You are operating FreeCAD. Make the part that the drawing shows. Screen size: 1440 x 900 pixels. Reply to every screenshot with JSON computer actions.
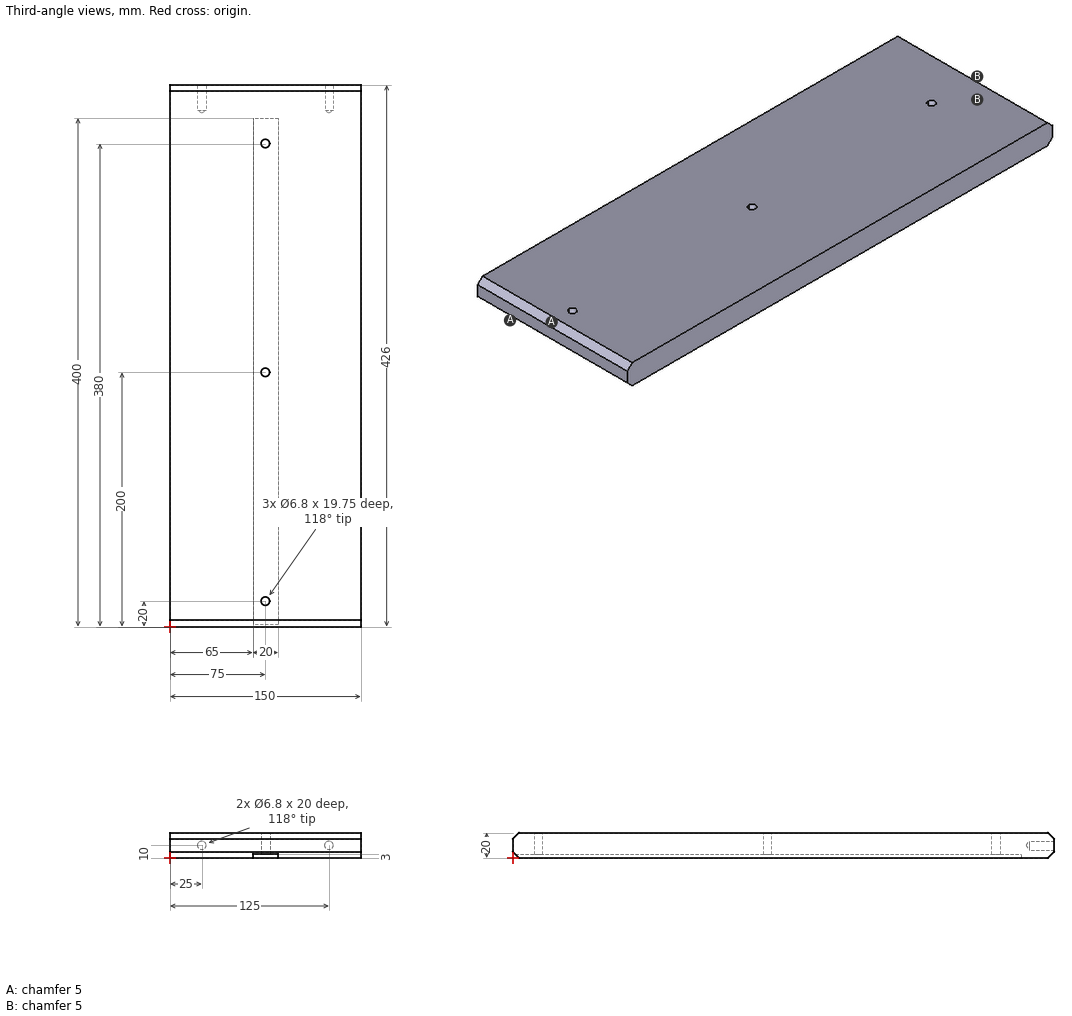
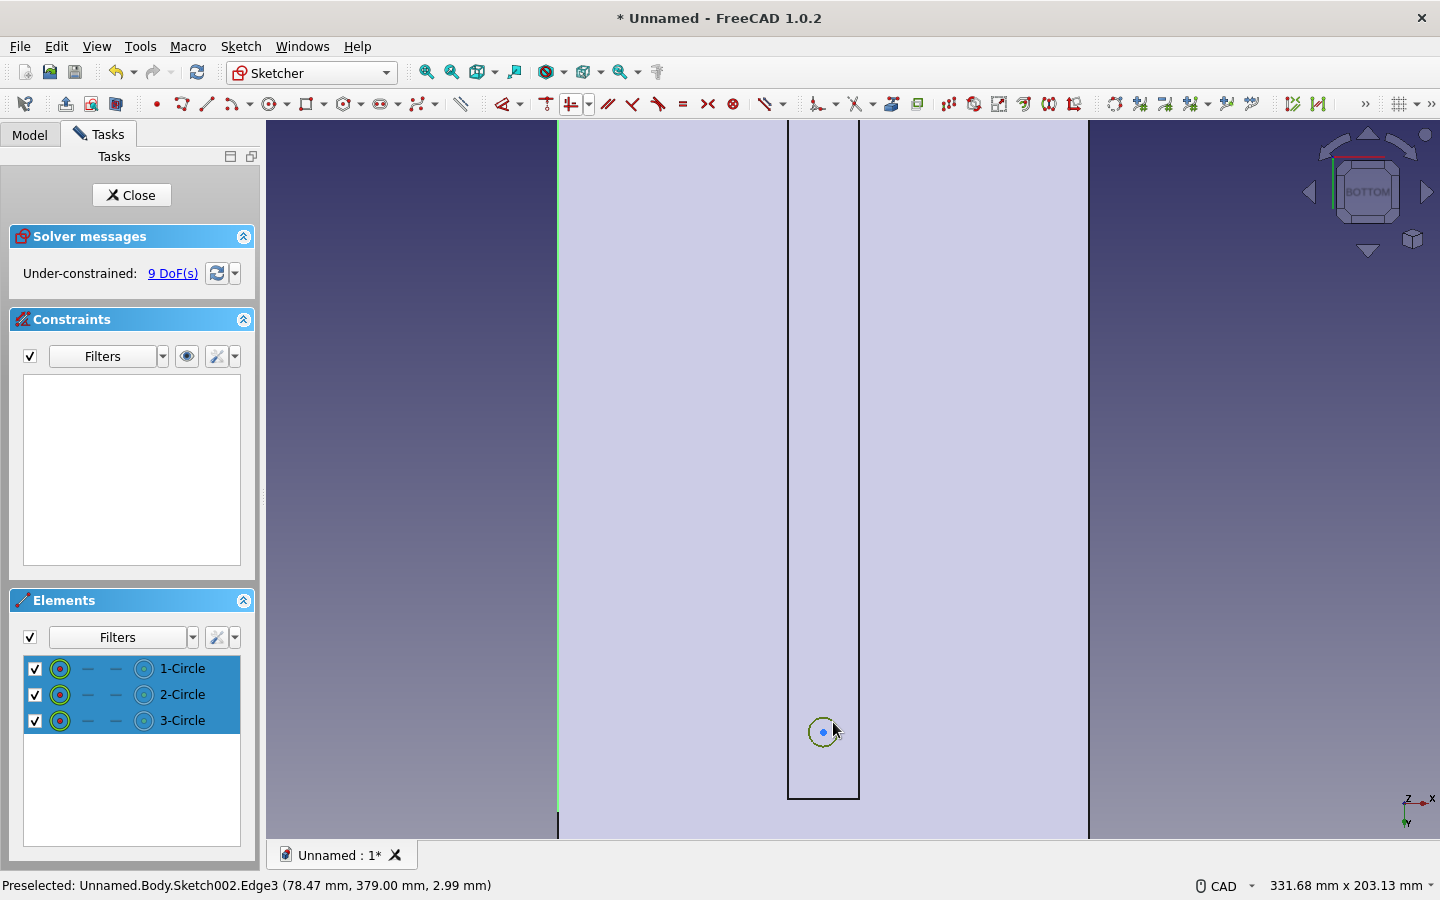
{"action": "left_click", "coordinate": [683, 104]}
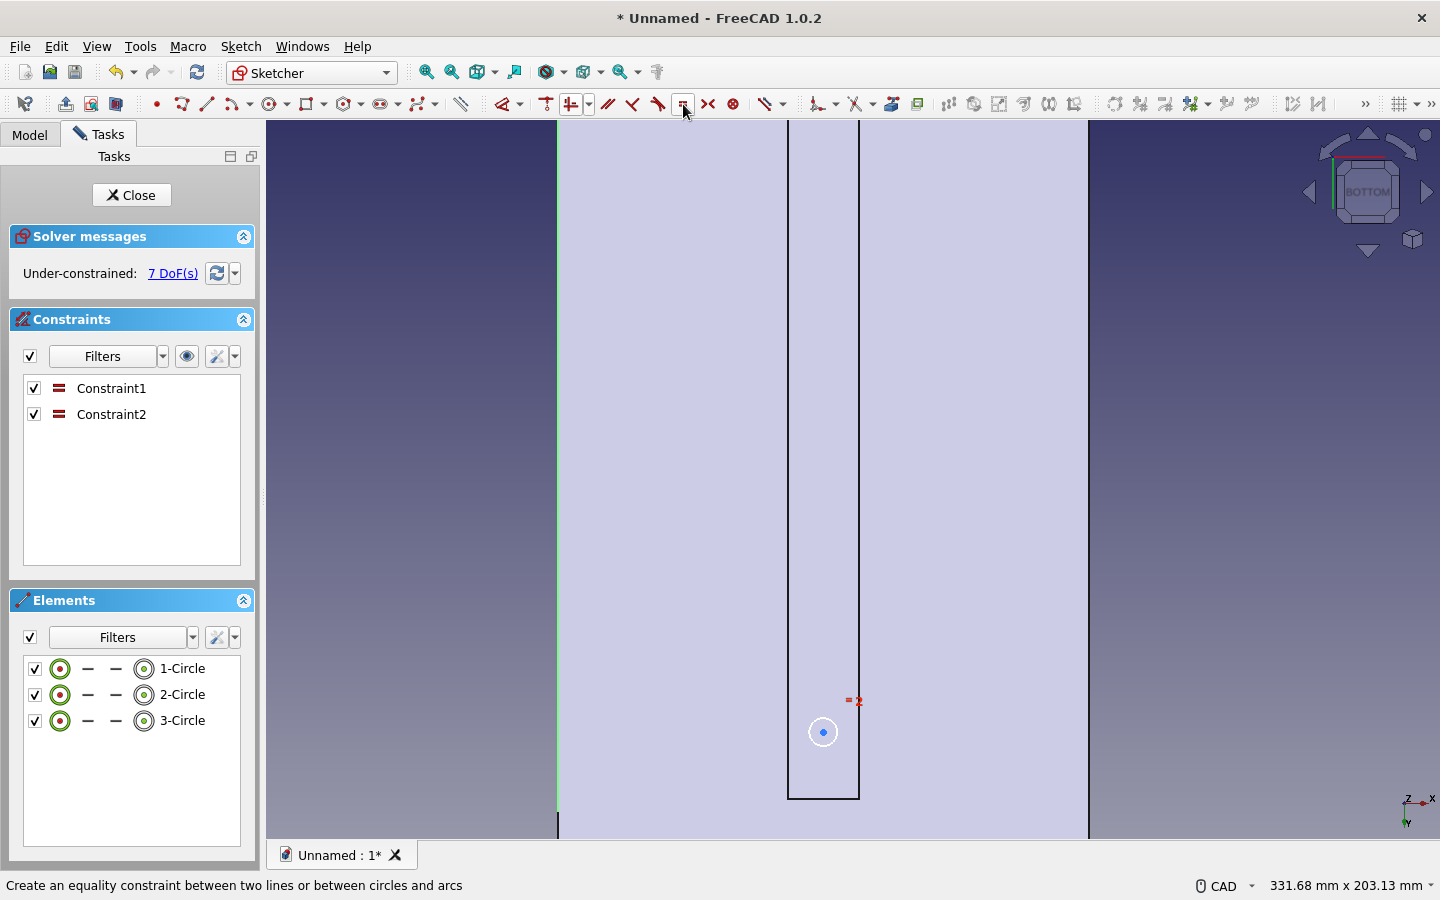
{"action": "scroll", "coordinate": [835, 722], "scroll_direction": "down", "scroll_amount": 5}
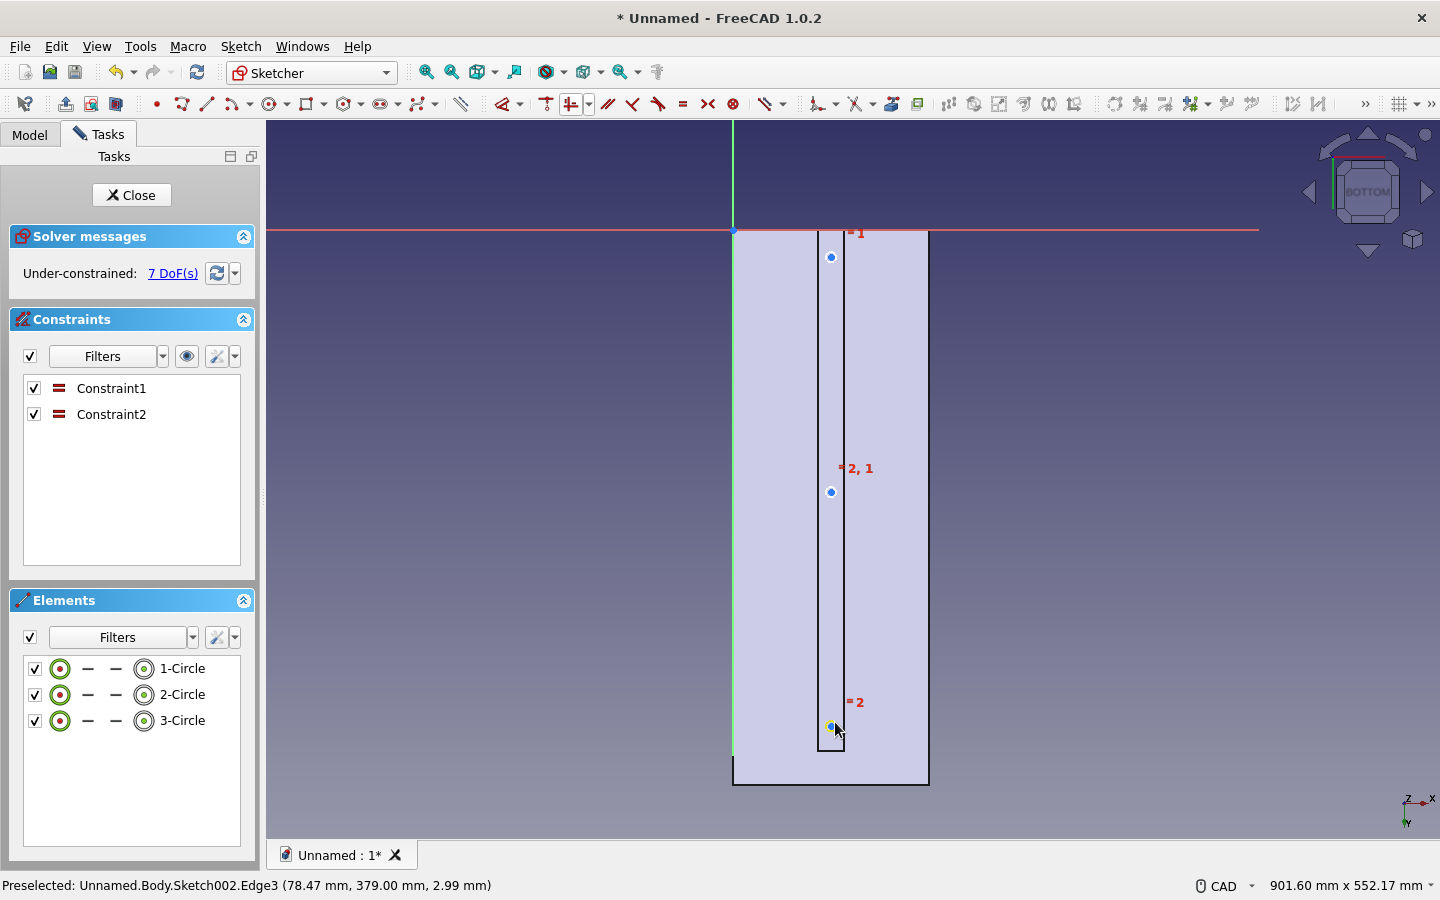
{"action": "left_click", "coordinate": [831, 257]}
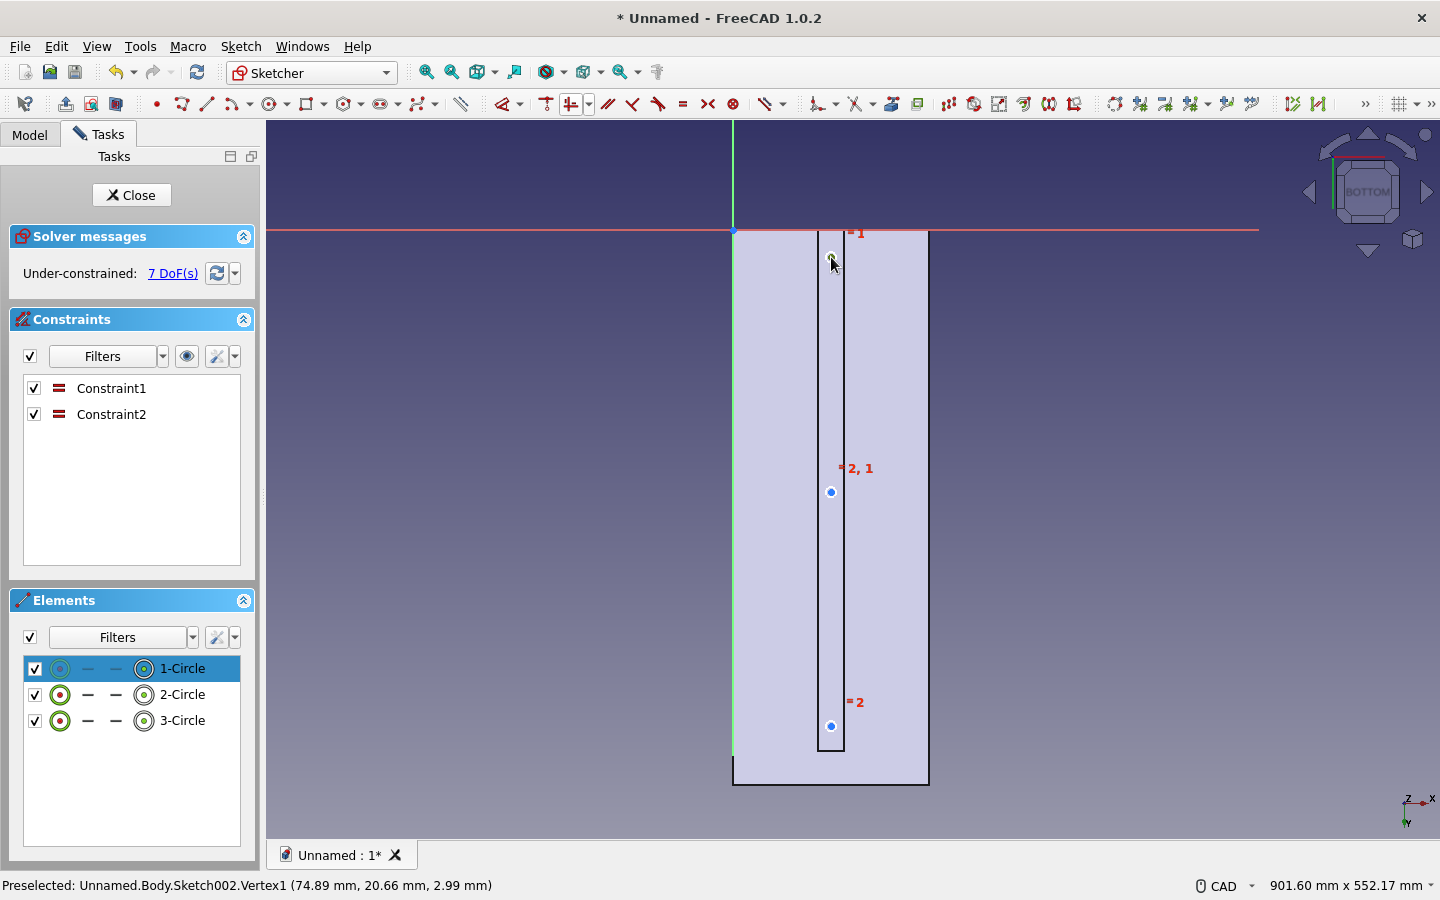
{"action": "left_click", "coordinate": [831, 492]}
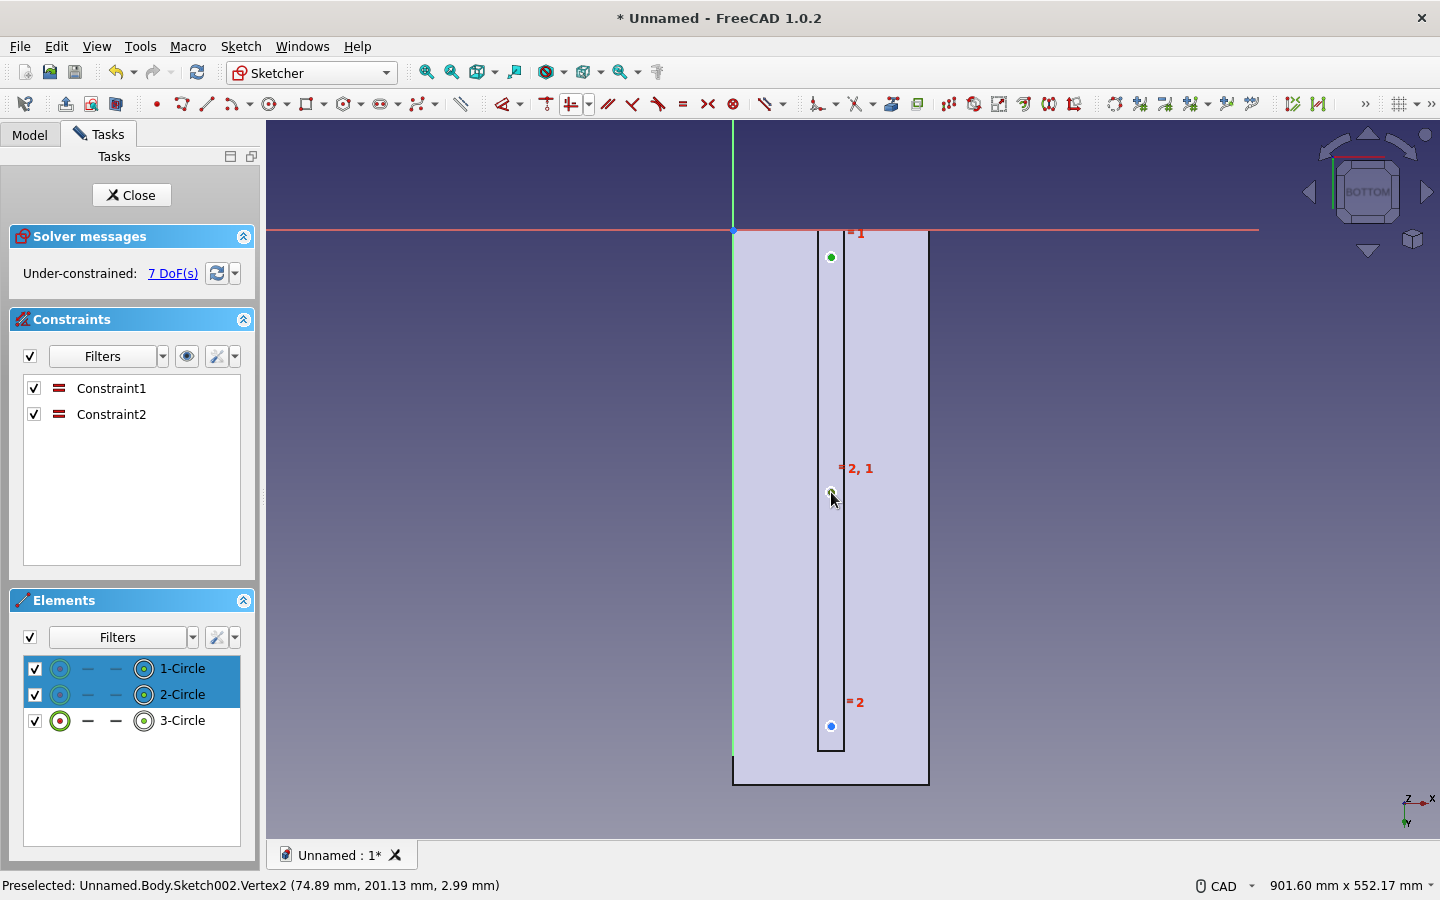
{"action": "left_click", "coordinate": [588, 104]}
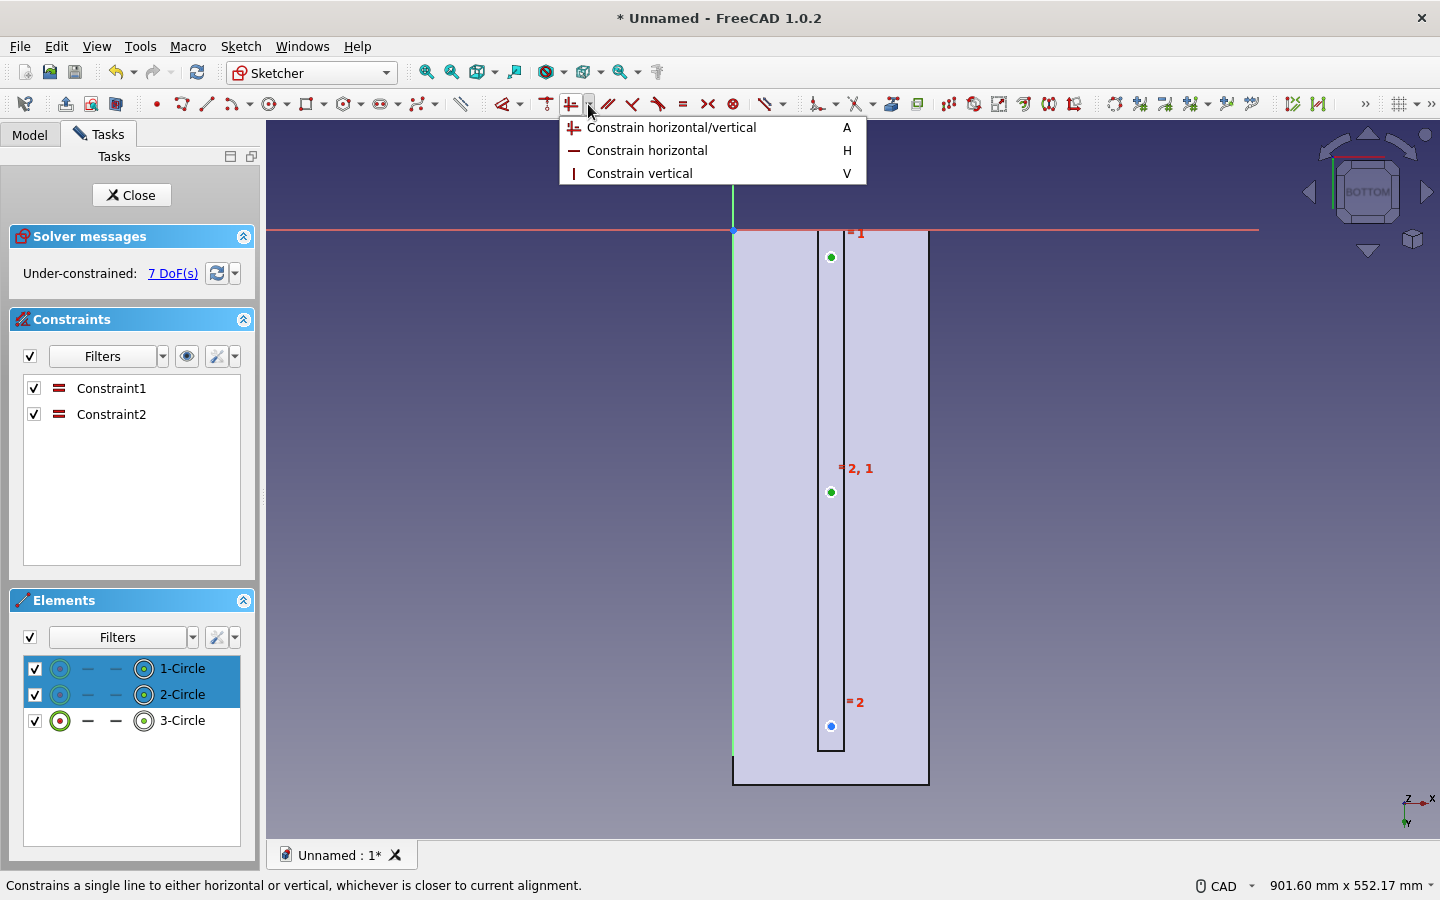
{"action": "left_click", "coordinate": [713, 174]}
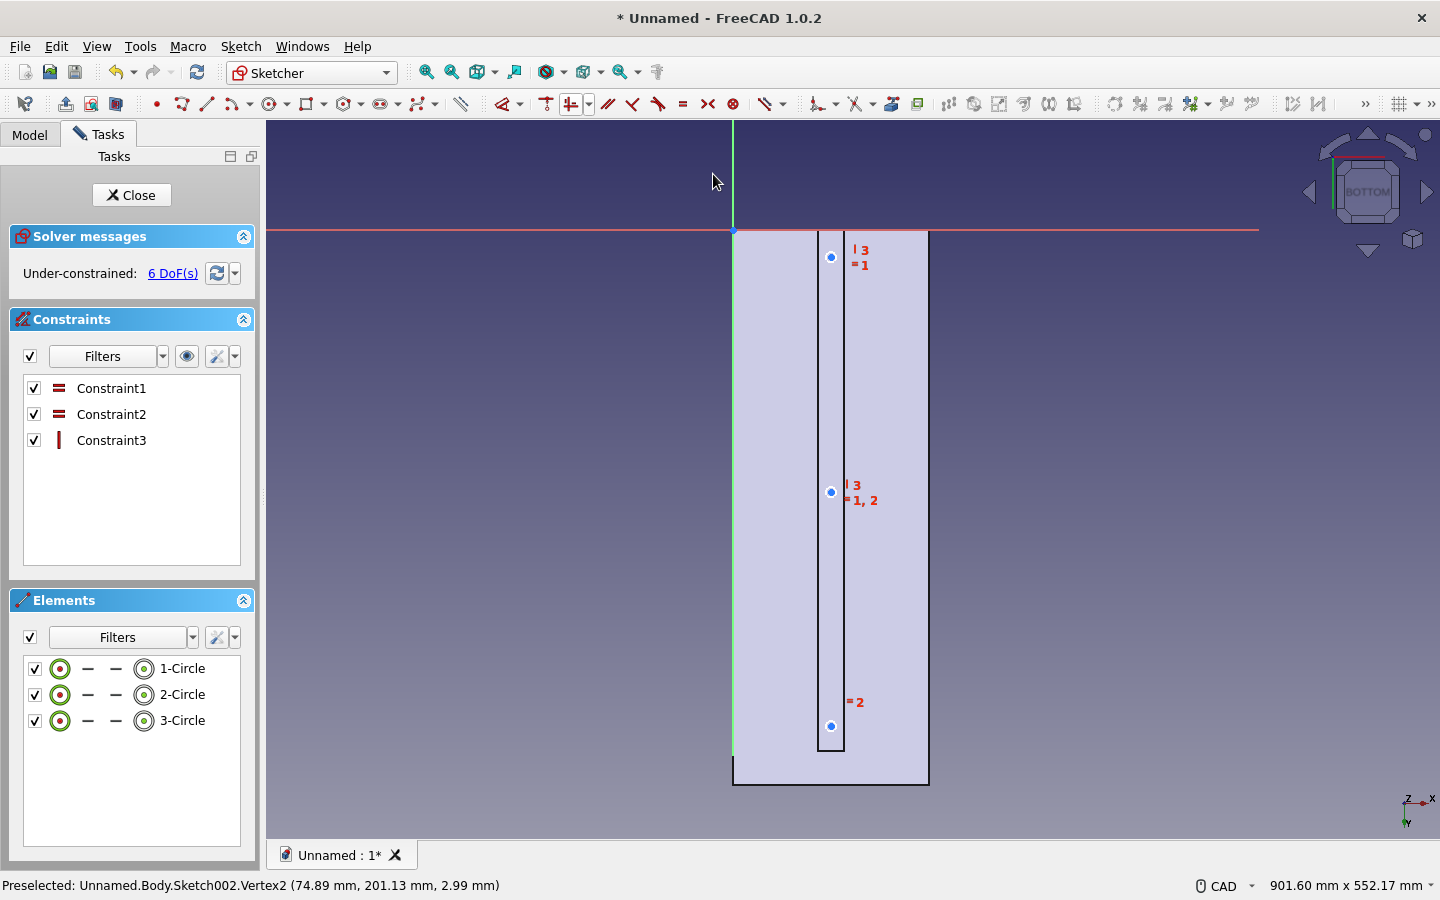
{"action": "left_click", "coordinate": [831, 492]}